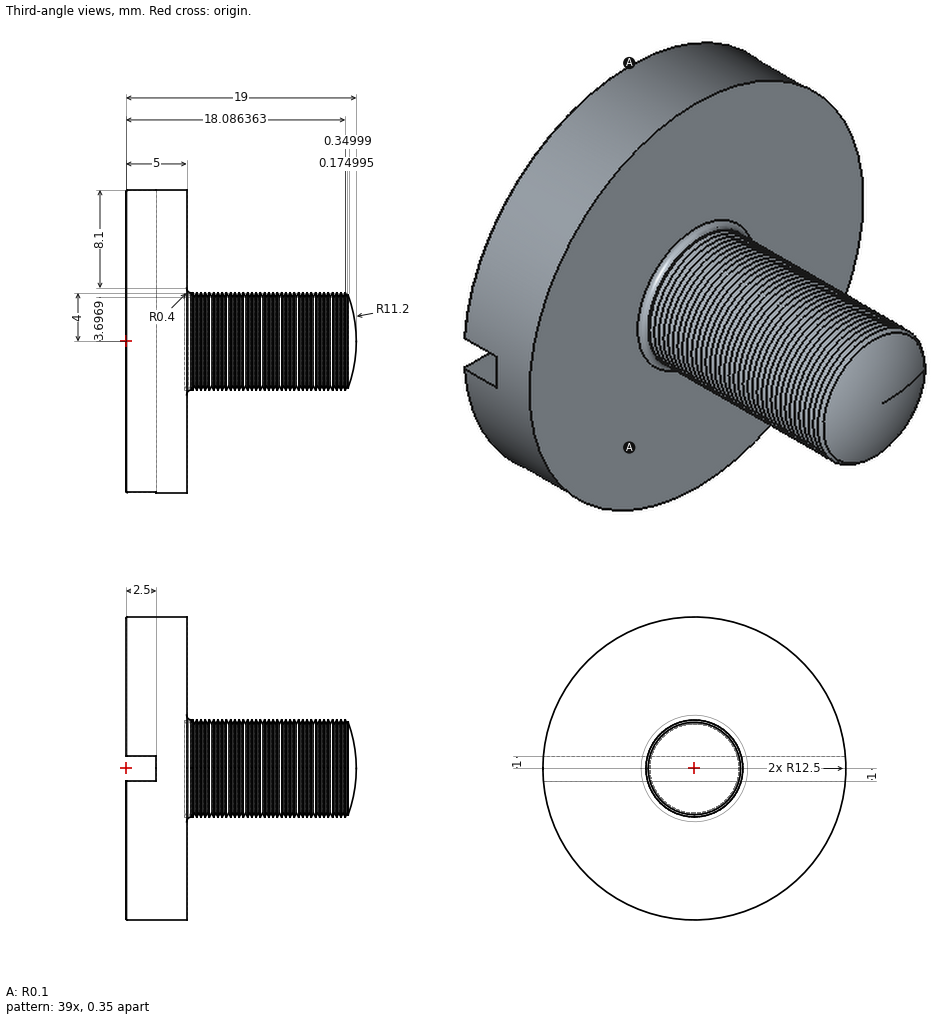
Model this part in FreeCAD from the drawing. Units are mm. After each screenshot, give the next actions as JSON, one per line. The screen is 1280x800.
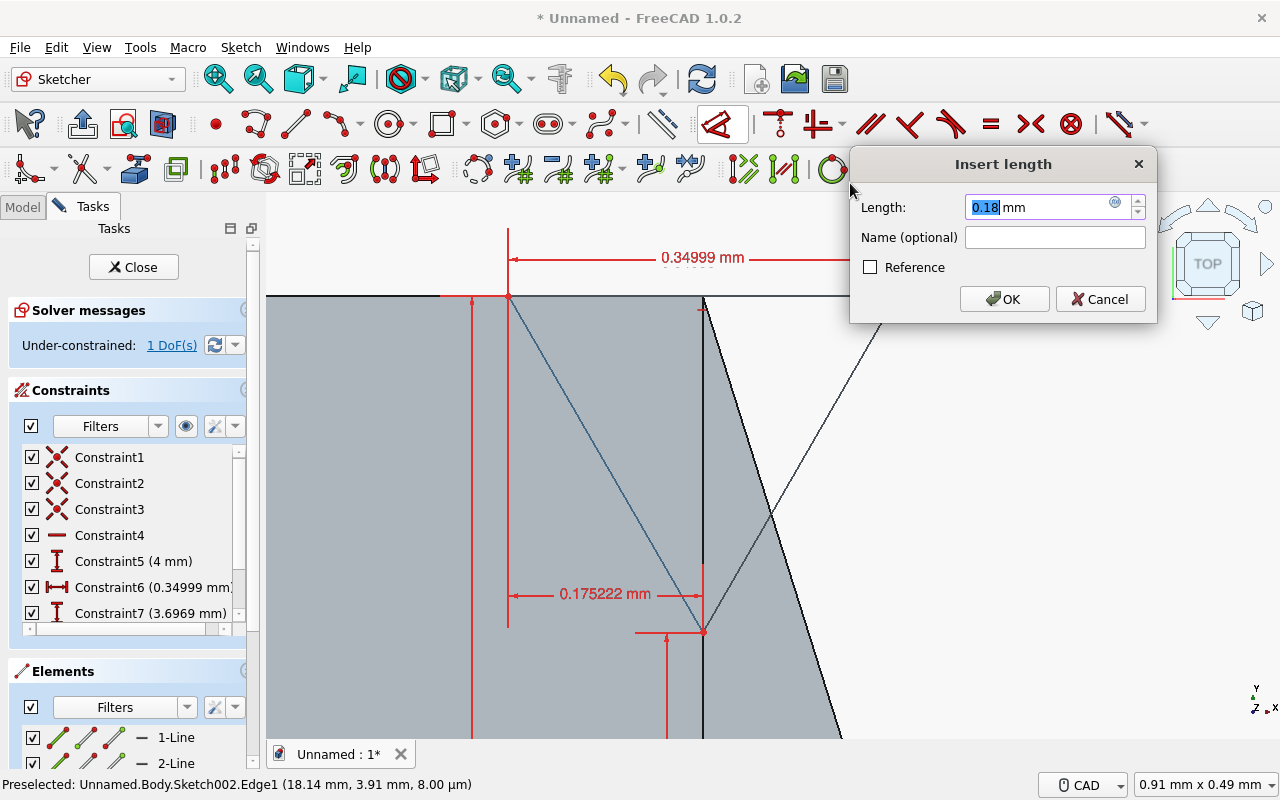
{"action": "type", "text": "0.174995"}
{"action": "key", "text": "Return"}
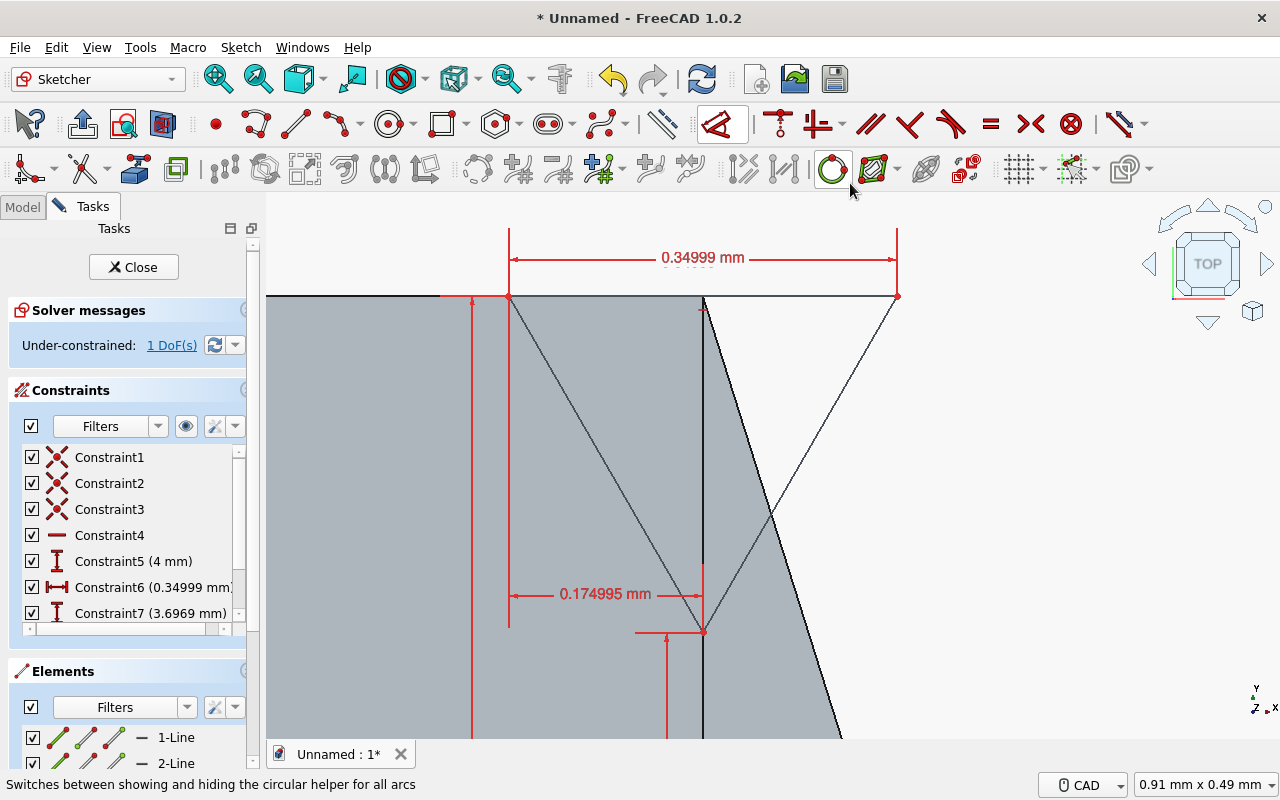
{"action": "left_click", "coordinate": [509, 296]}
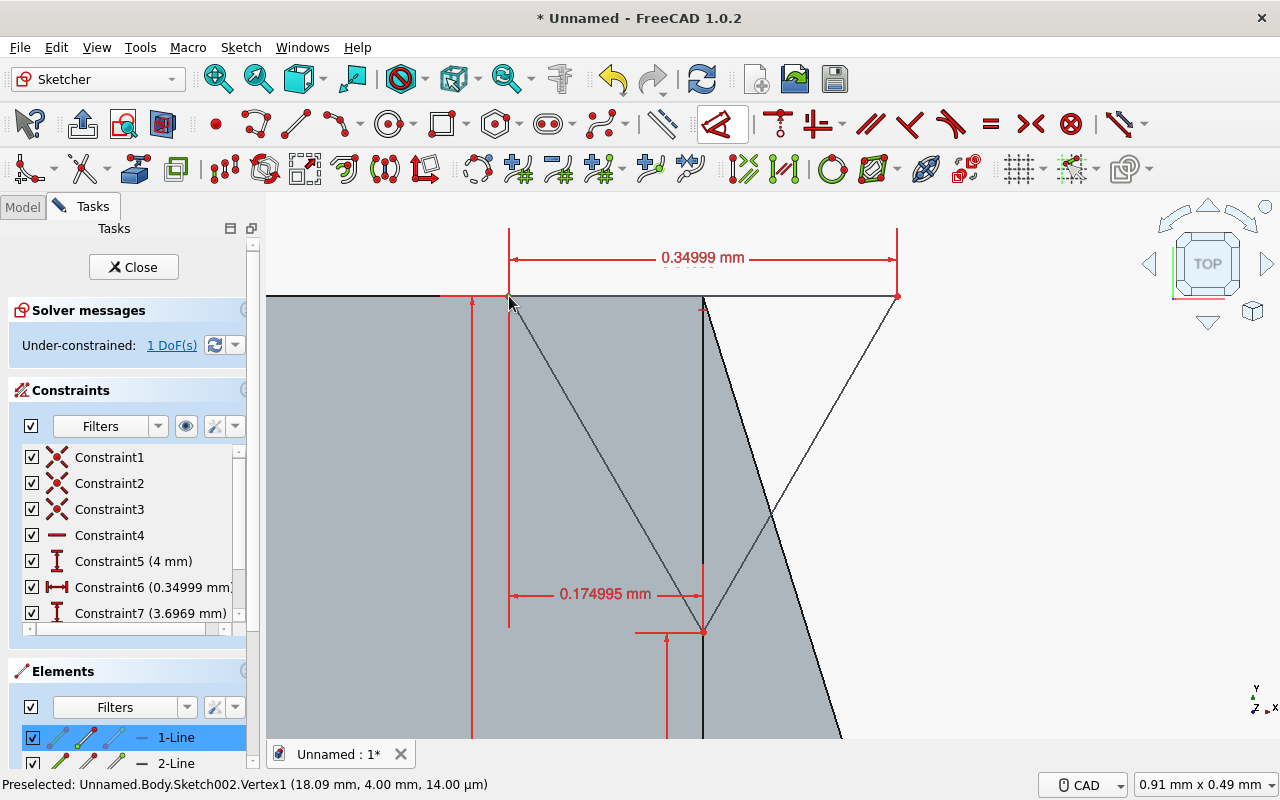
{"action": "left_click", "coordinate": [742, 124]}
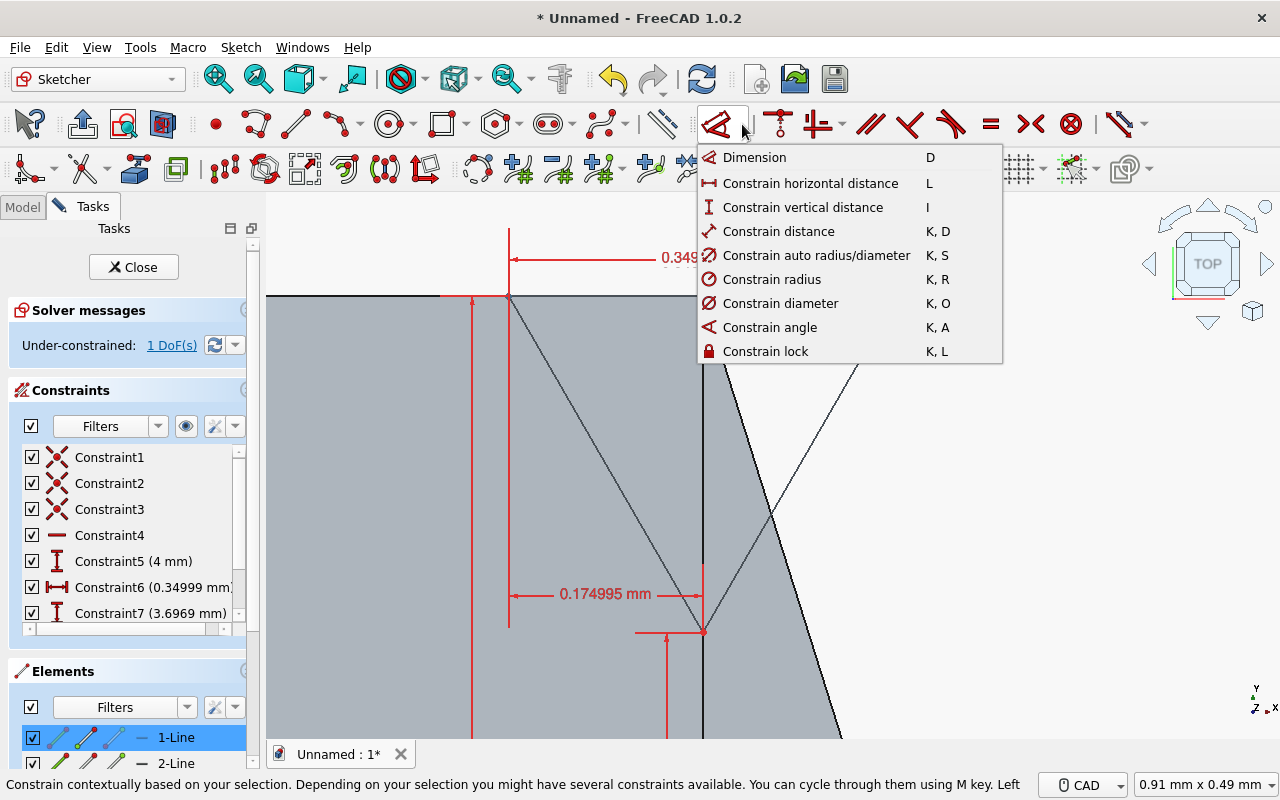
{"action": "left_click", "coordinate": [850, 183]}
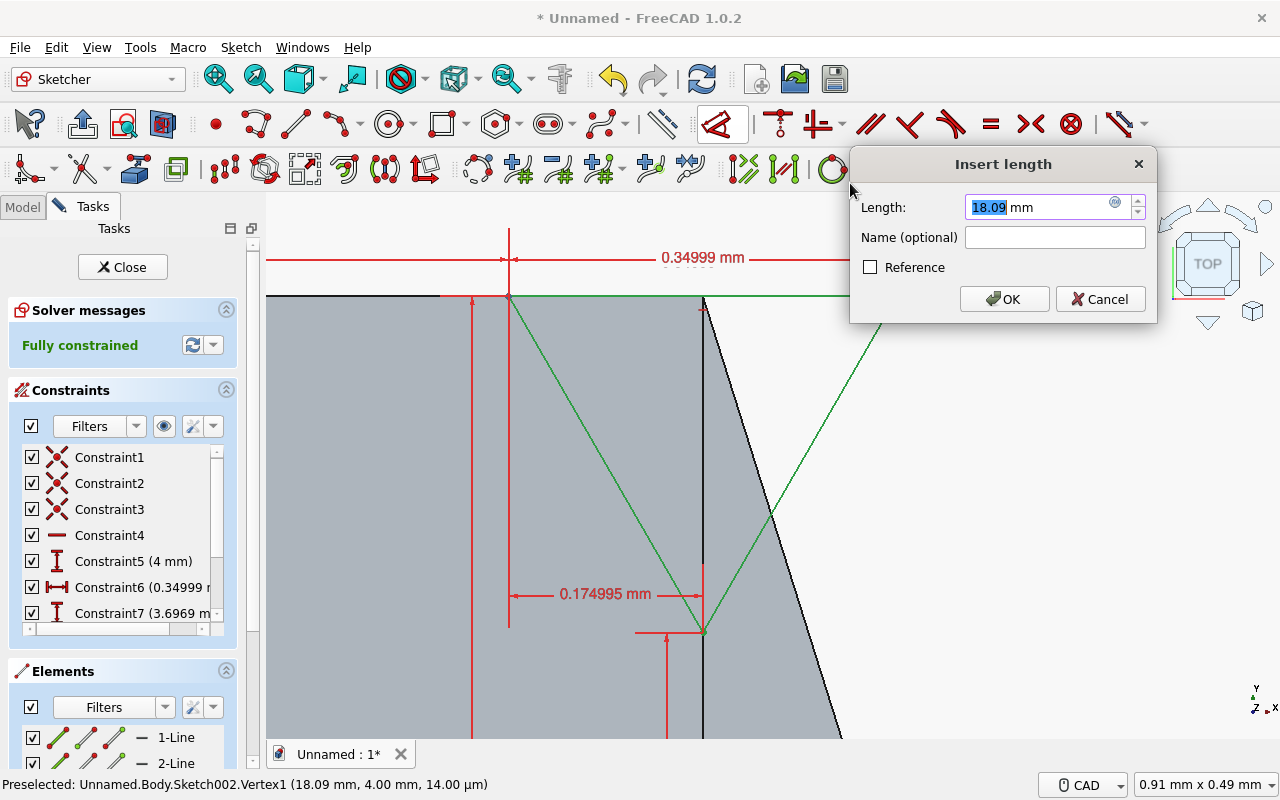
{"action": "type", "text": "18.086363"}
{"action": "key", "text": "Return"}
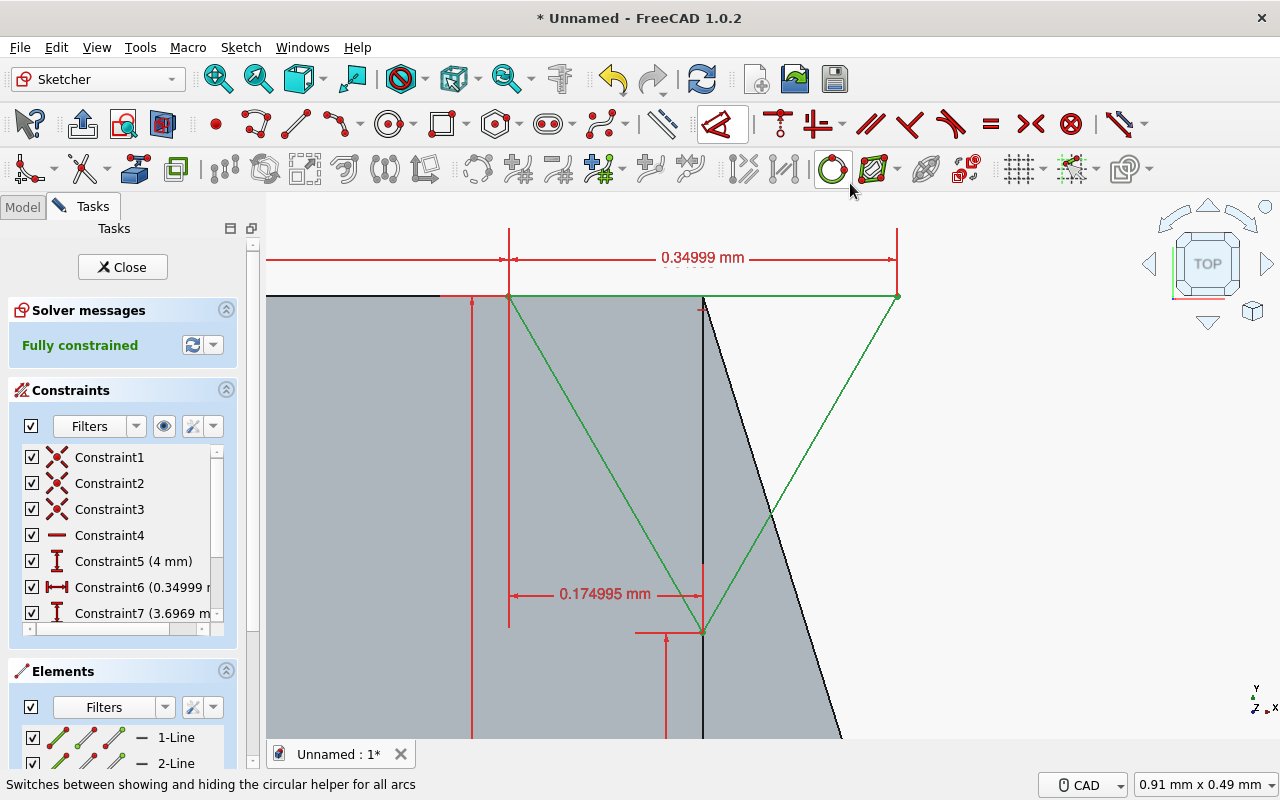
{"action": "left_click", "coordinate": [123, 267]}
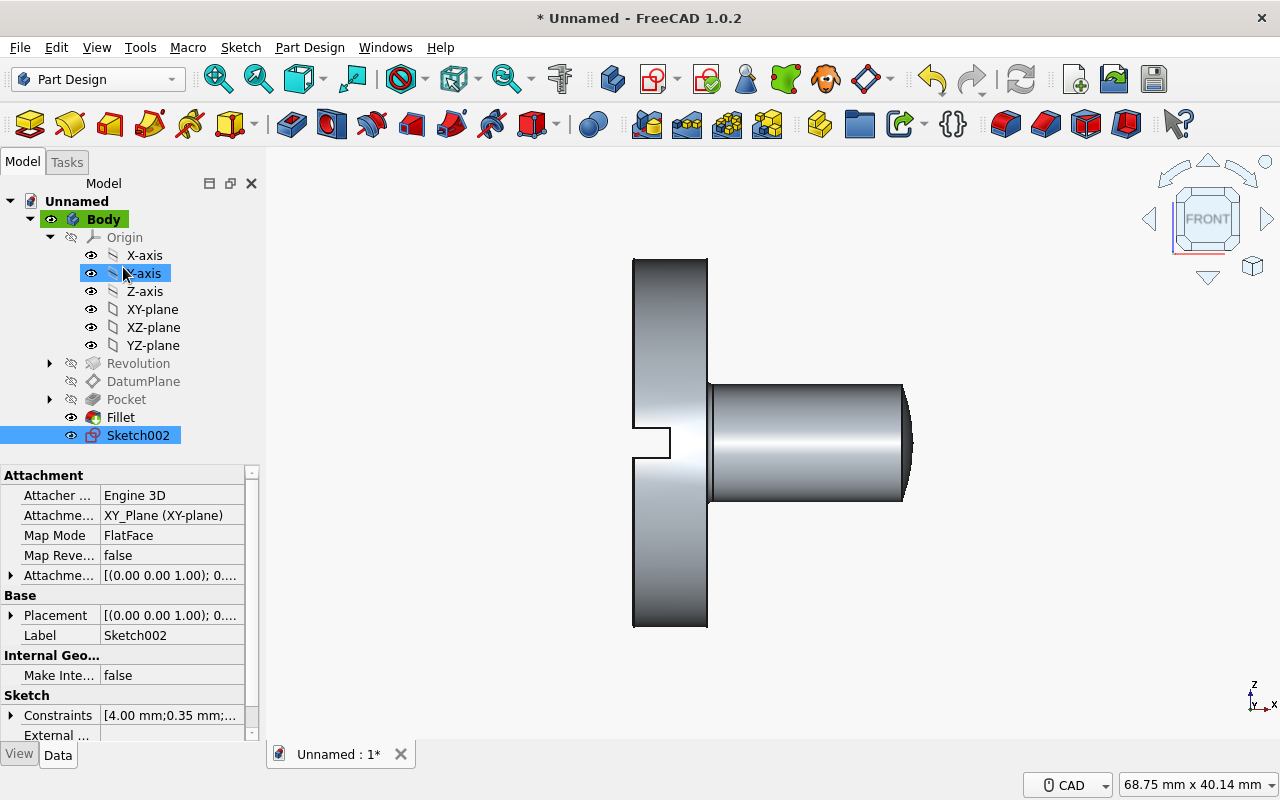
{"action": "left_click", "coordinate": [372, 124]}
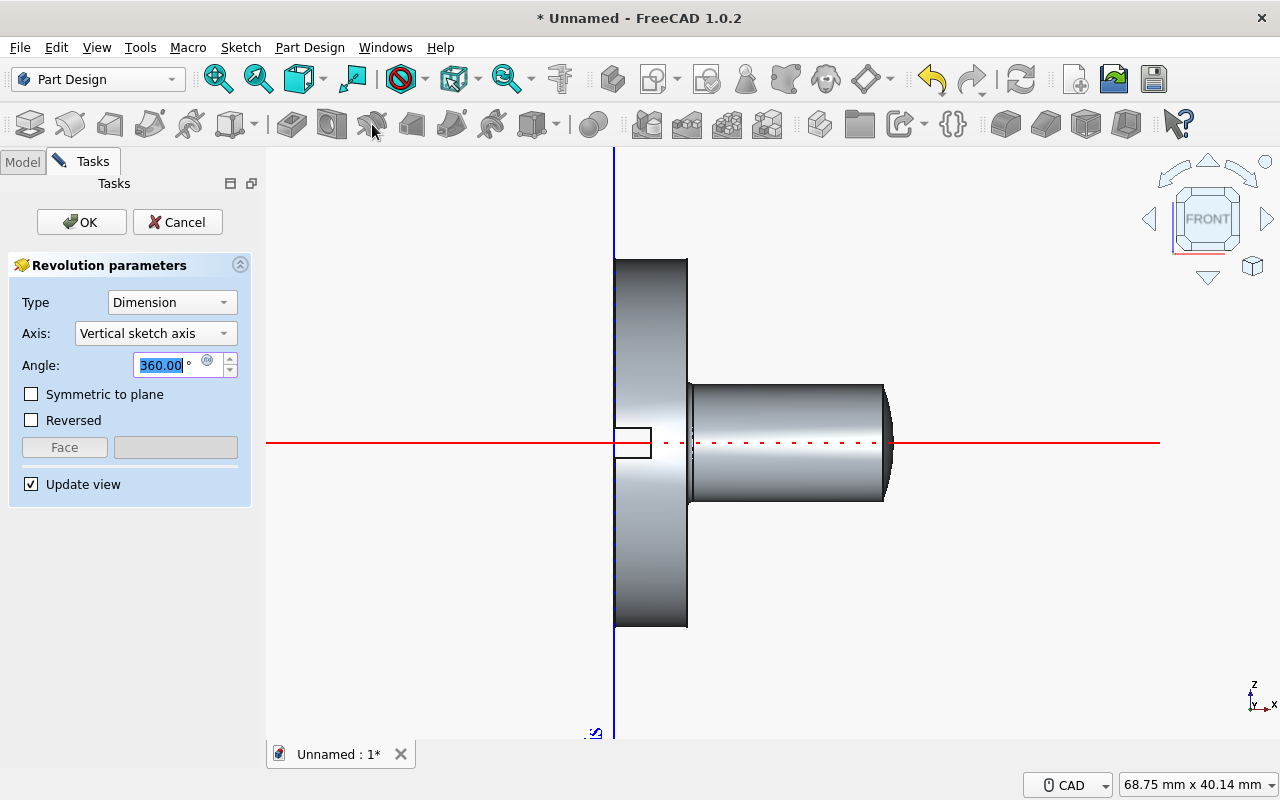
{"action": "left_click", "coordinate": [156, 334]}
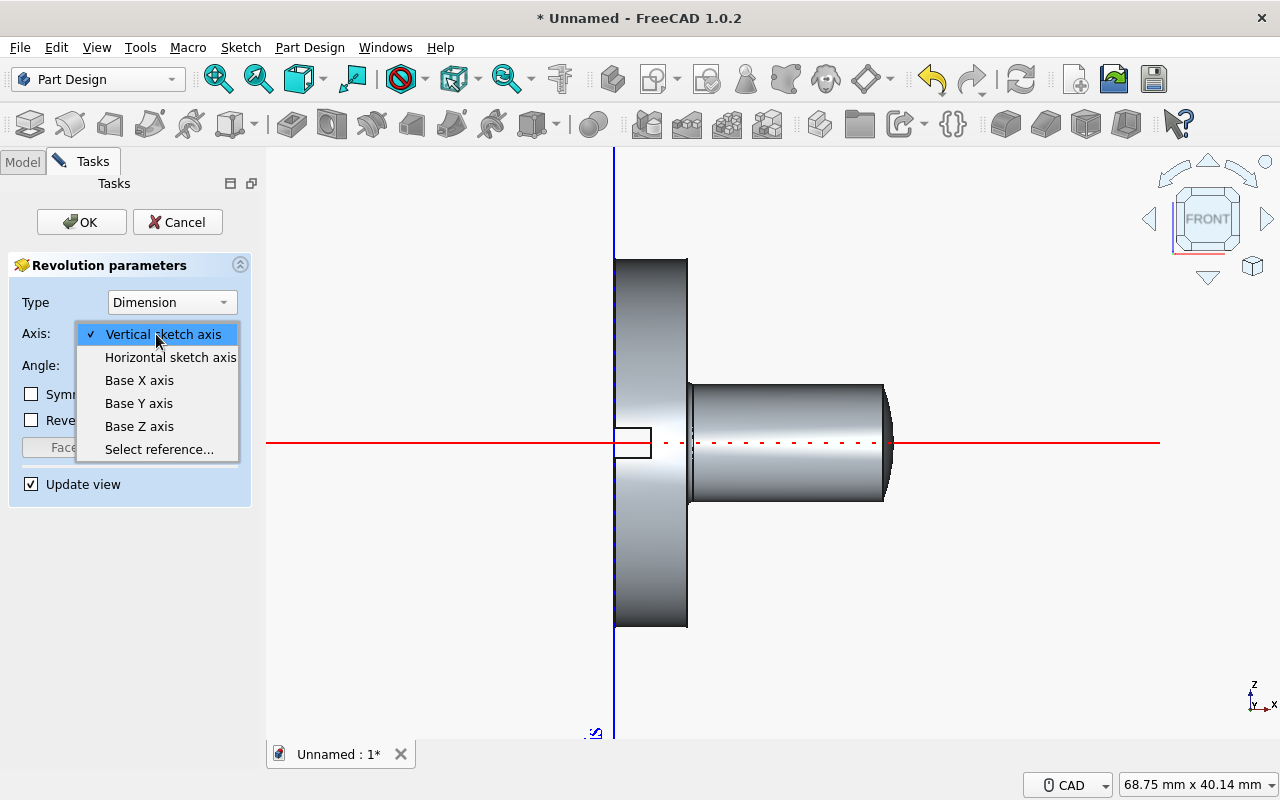
{"action": "left_click", "coordinate": [156, 358]}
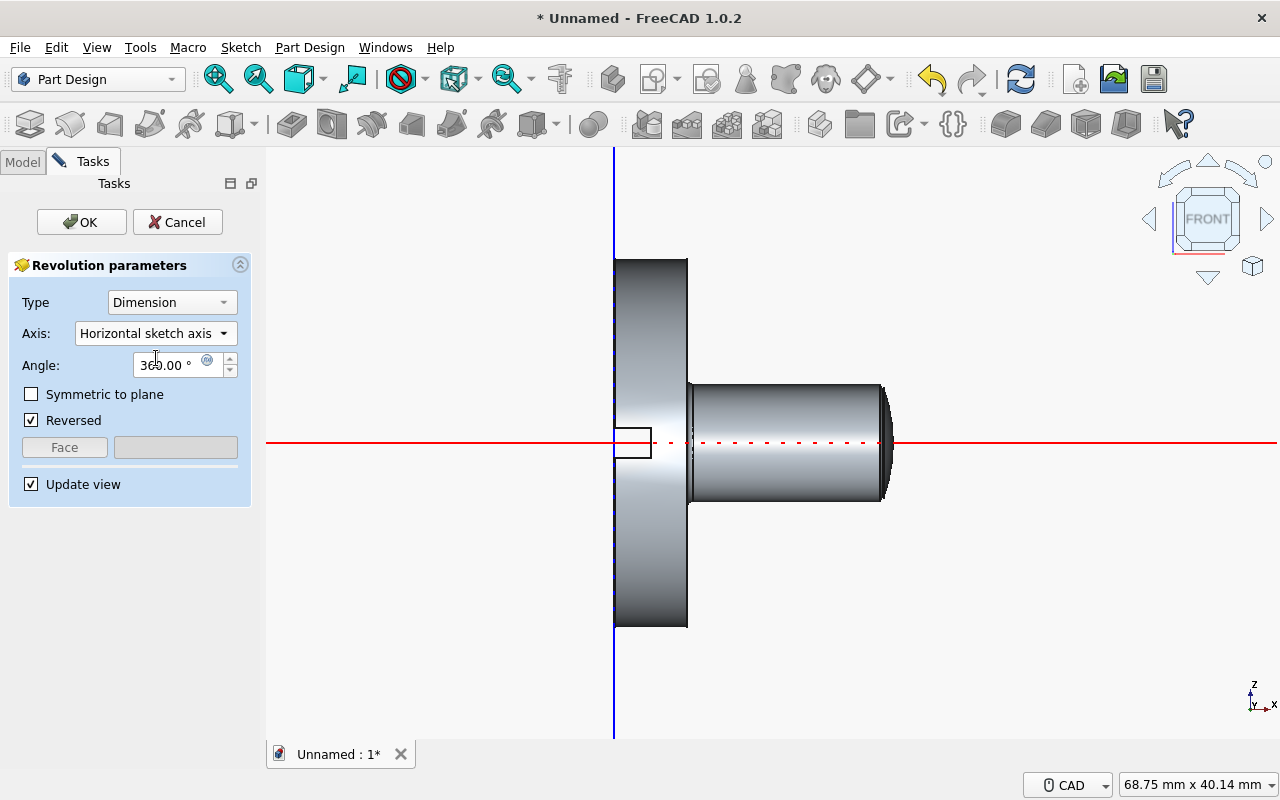
{"action": "left_click", "coordinate": [82, 222]}